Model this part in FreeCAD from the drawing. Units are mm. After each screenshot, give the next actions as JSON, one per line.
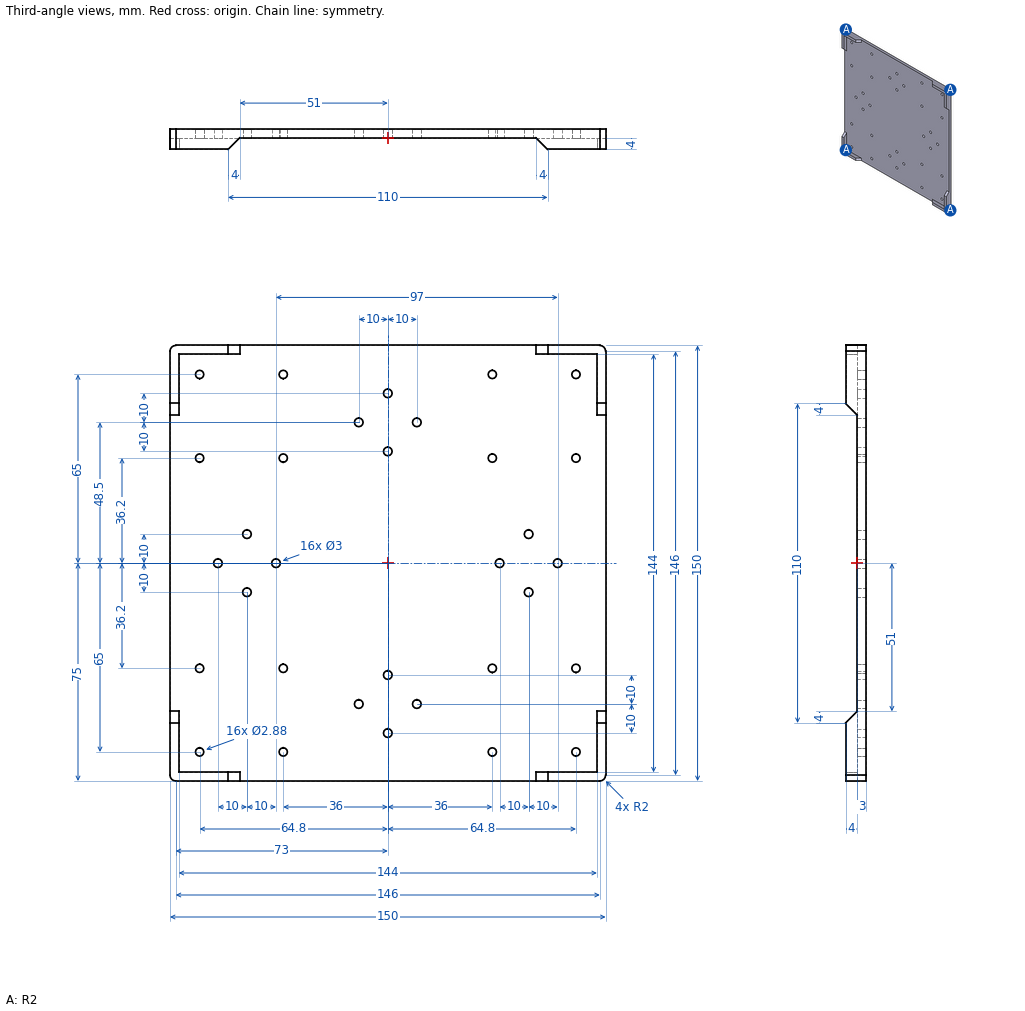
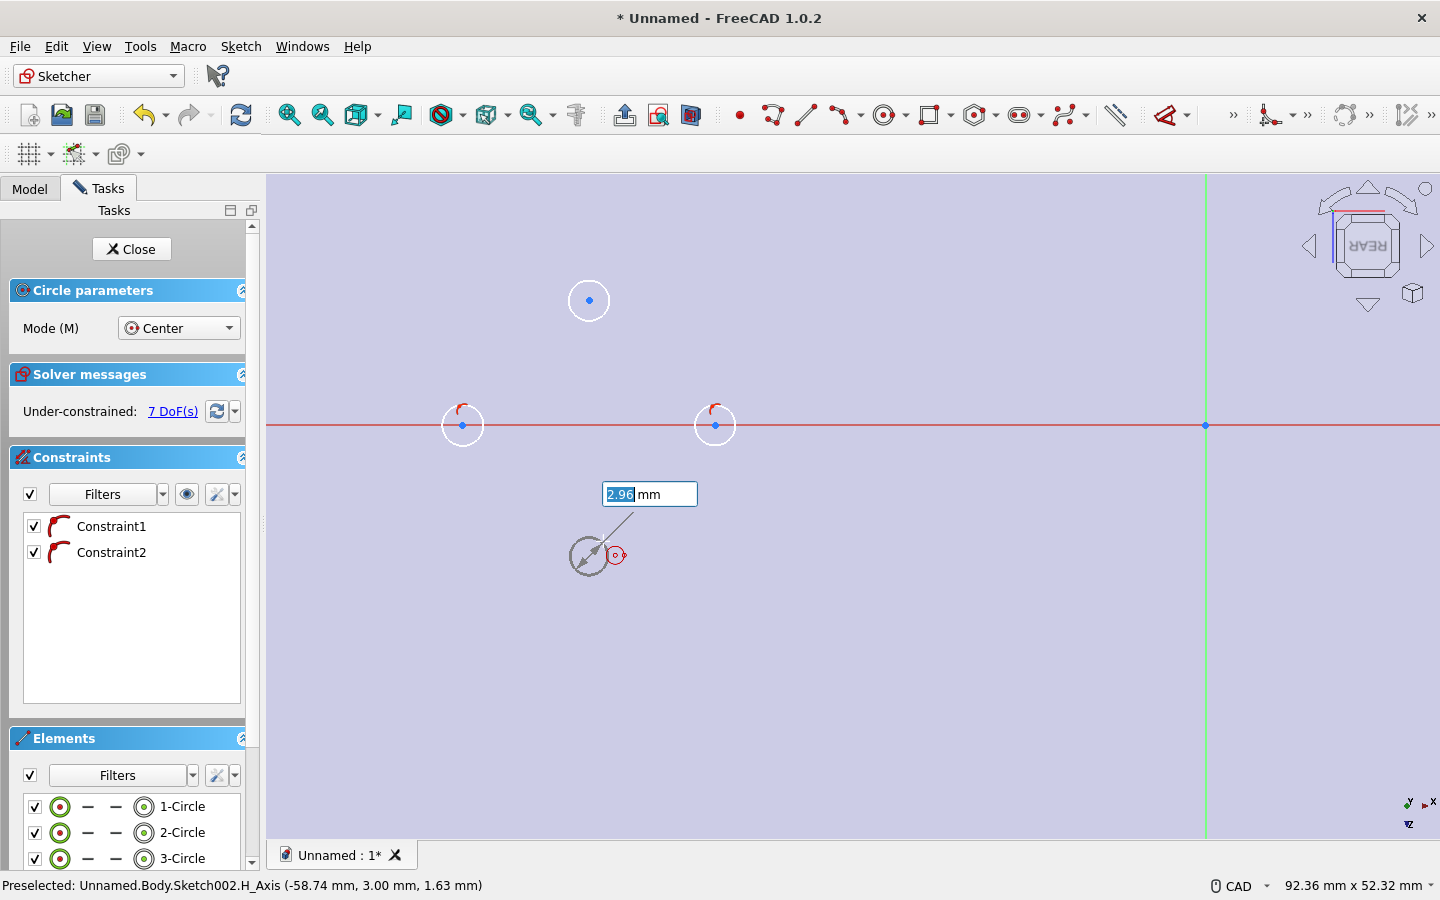
{"action": "left_click", "coordinate": [603, 539]}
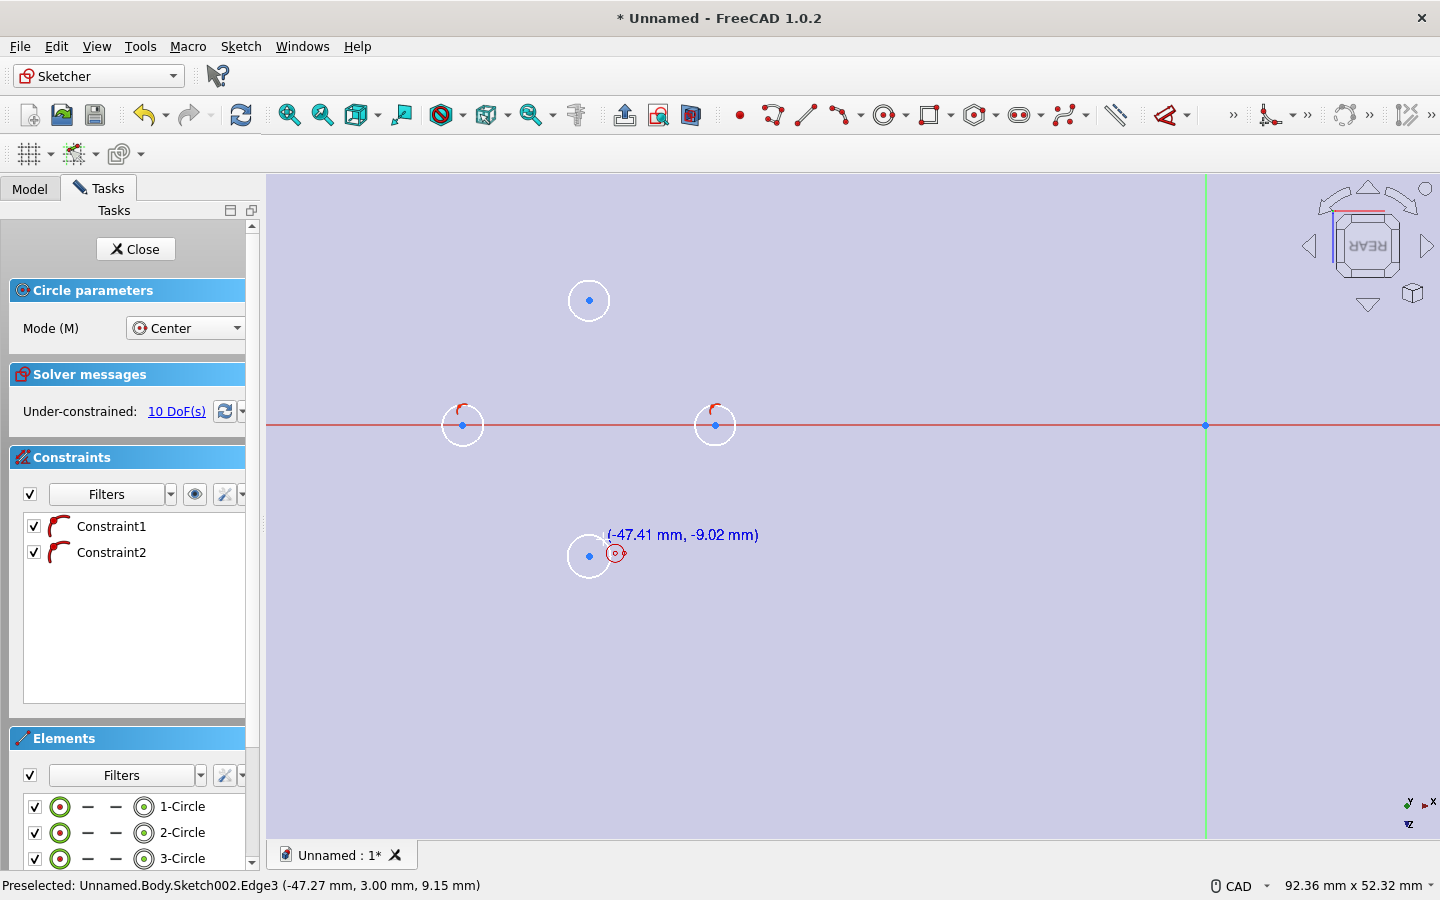
{"action": "scroll", "coordinate": [603, 541], "scroll_direction": "down", "scroll_amount": 6}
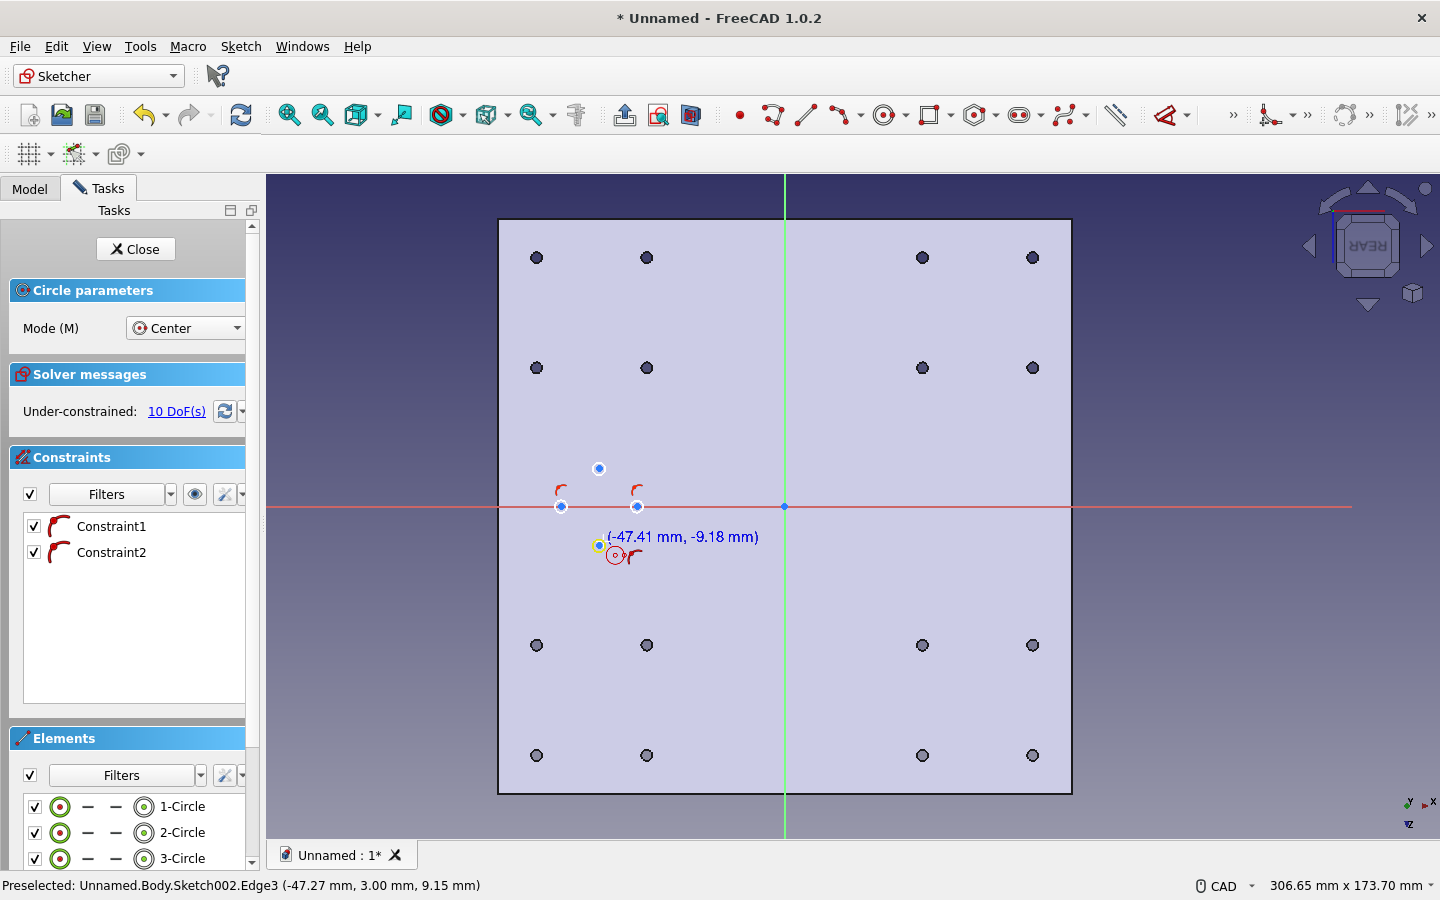
{"action": "scroll", "coordinate": [746, 692], "scroll_direction": "up", "scroll_amount": 7}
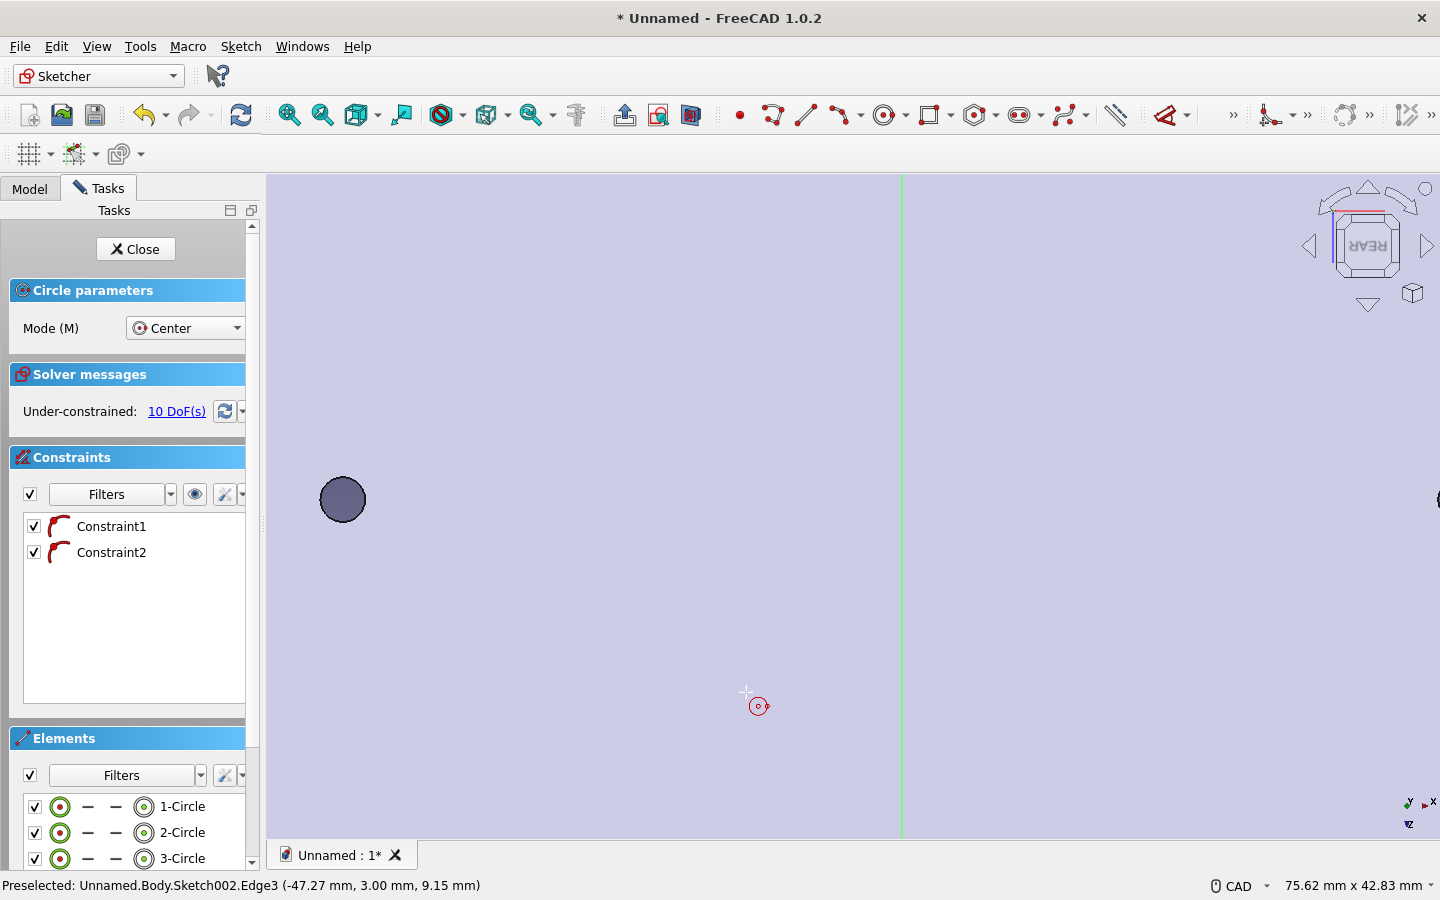
{"action": "scroll", "coordinate": [746, 693], "scroll_direction": "down", "scroll_amount": 7}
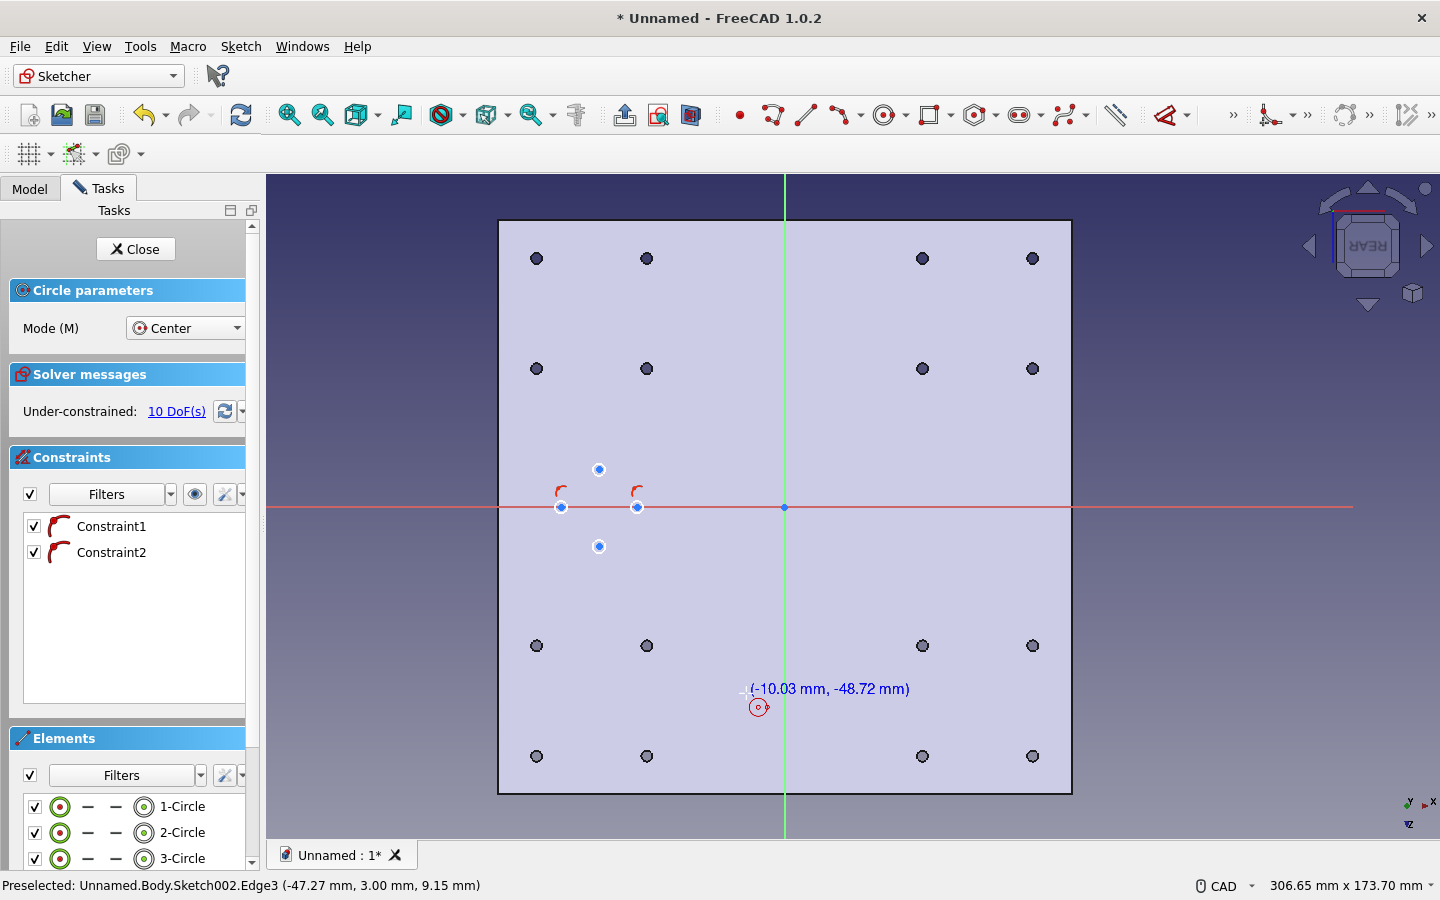
{"action": "left_click", "coordinate": [746, 693]}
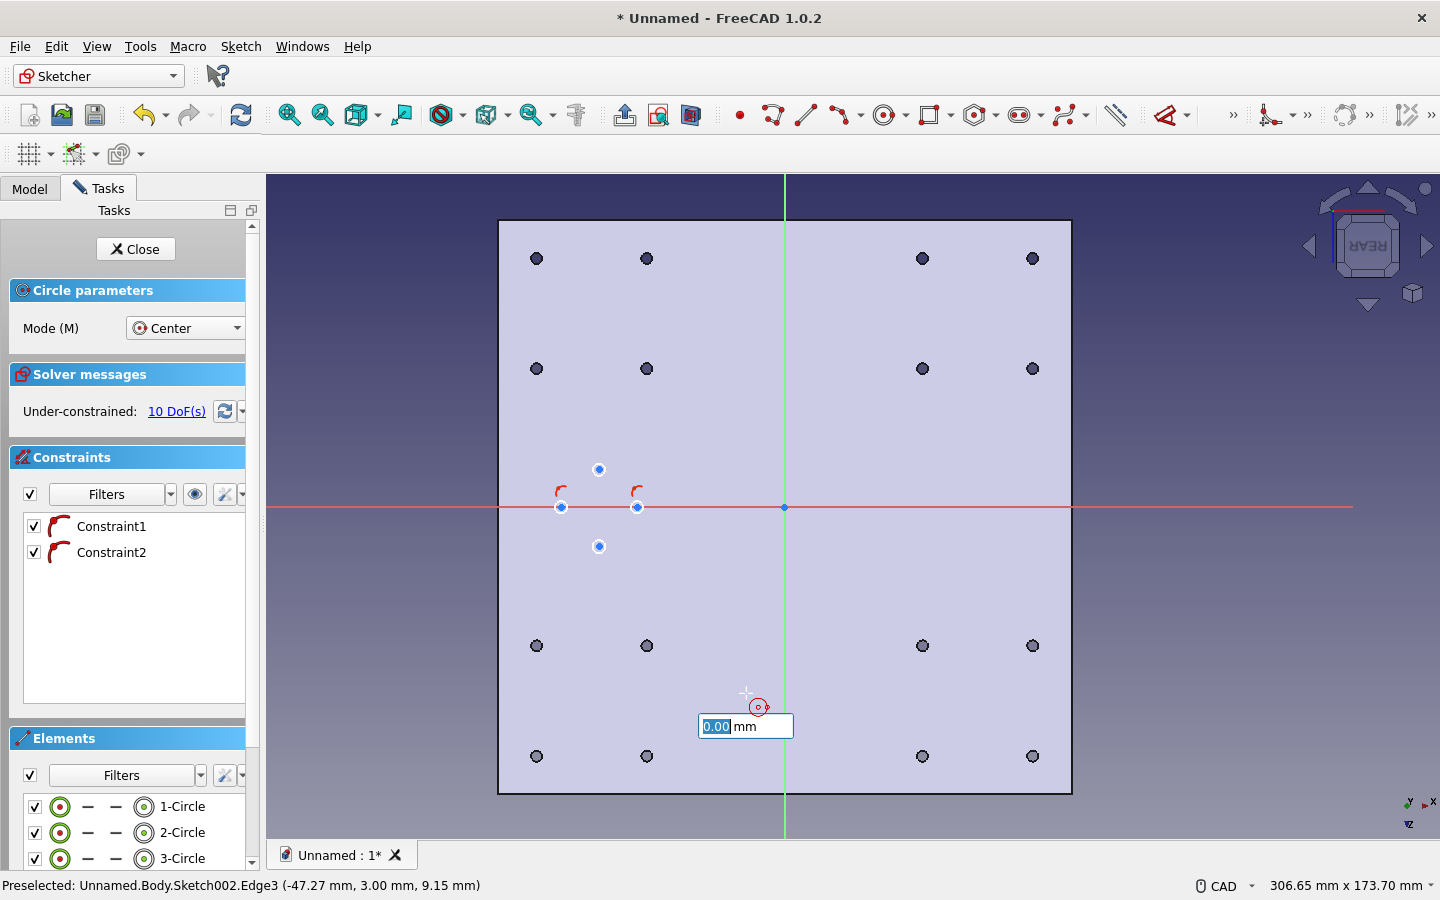
{"action": "scroll", "coordinate": [750, 689], "scroll_direction": "up", "scroll_amount": 6}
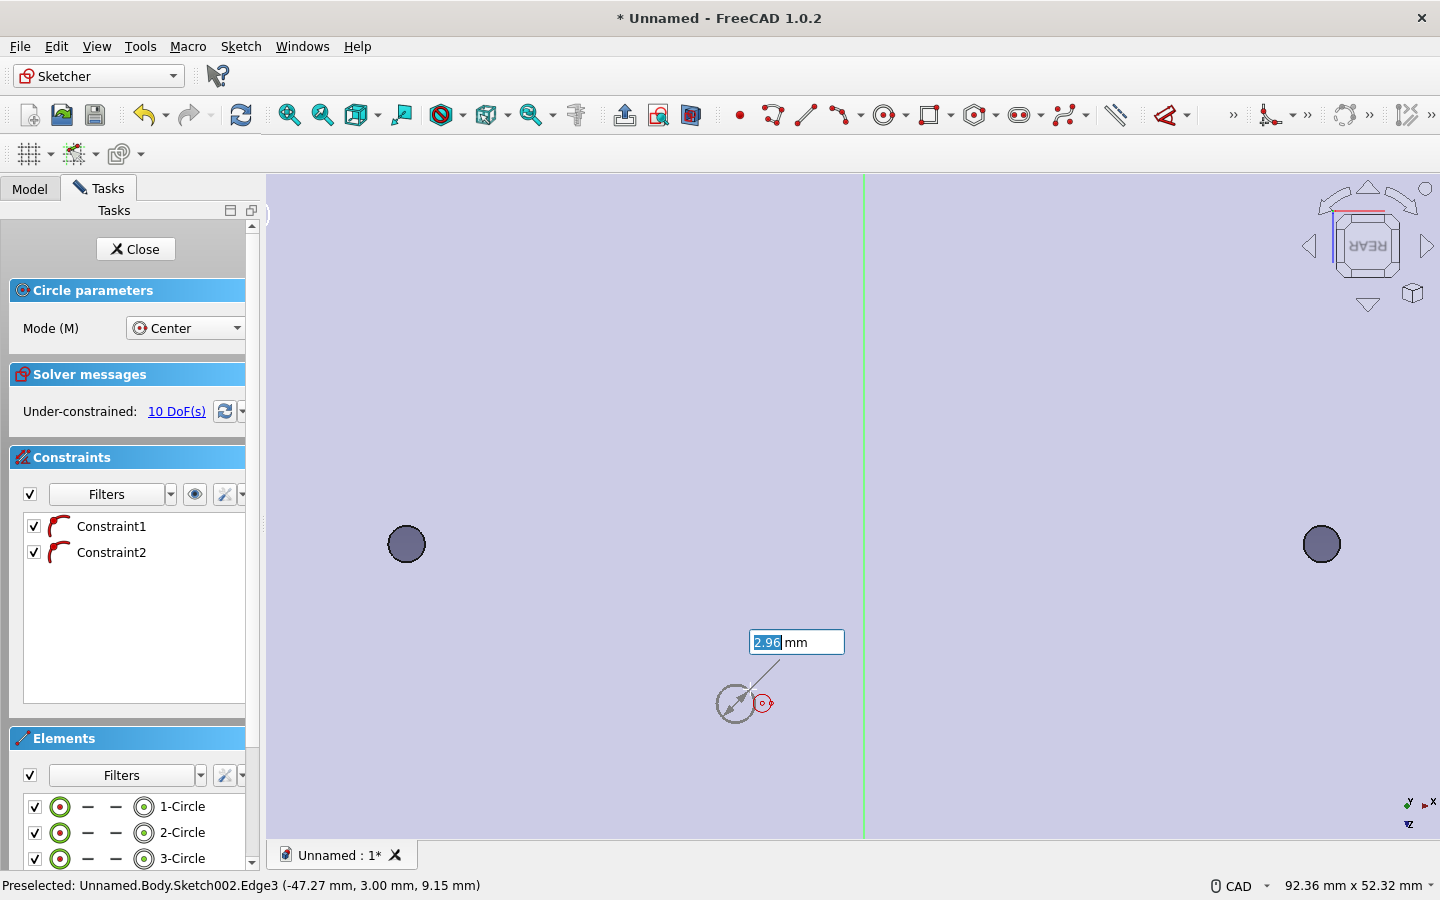
{"action": "left_click", "coordinate": [751, 687]}